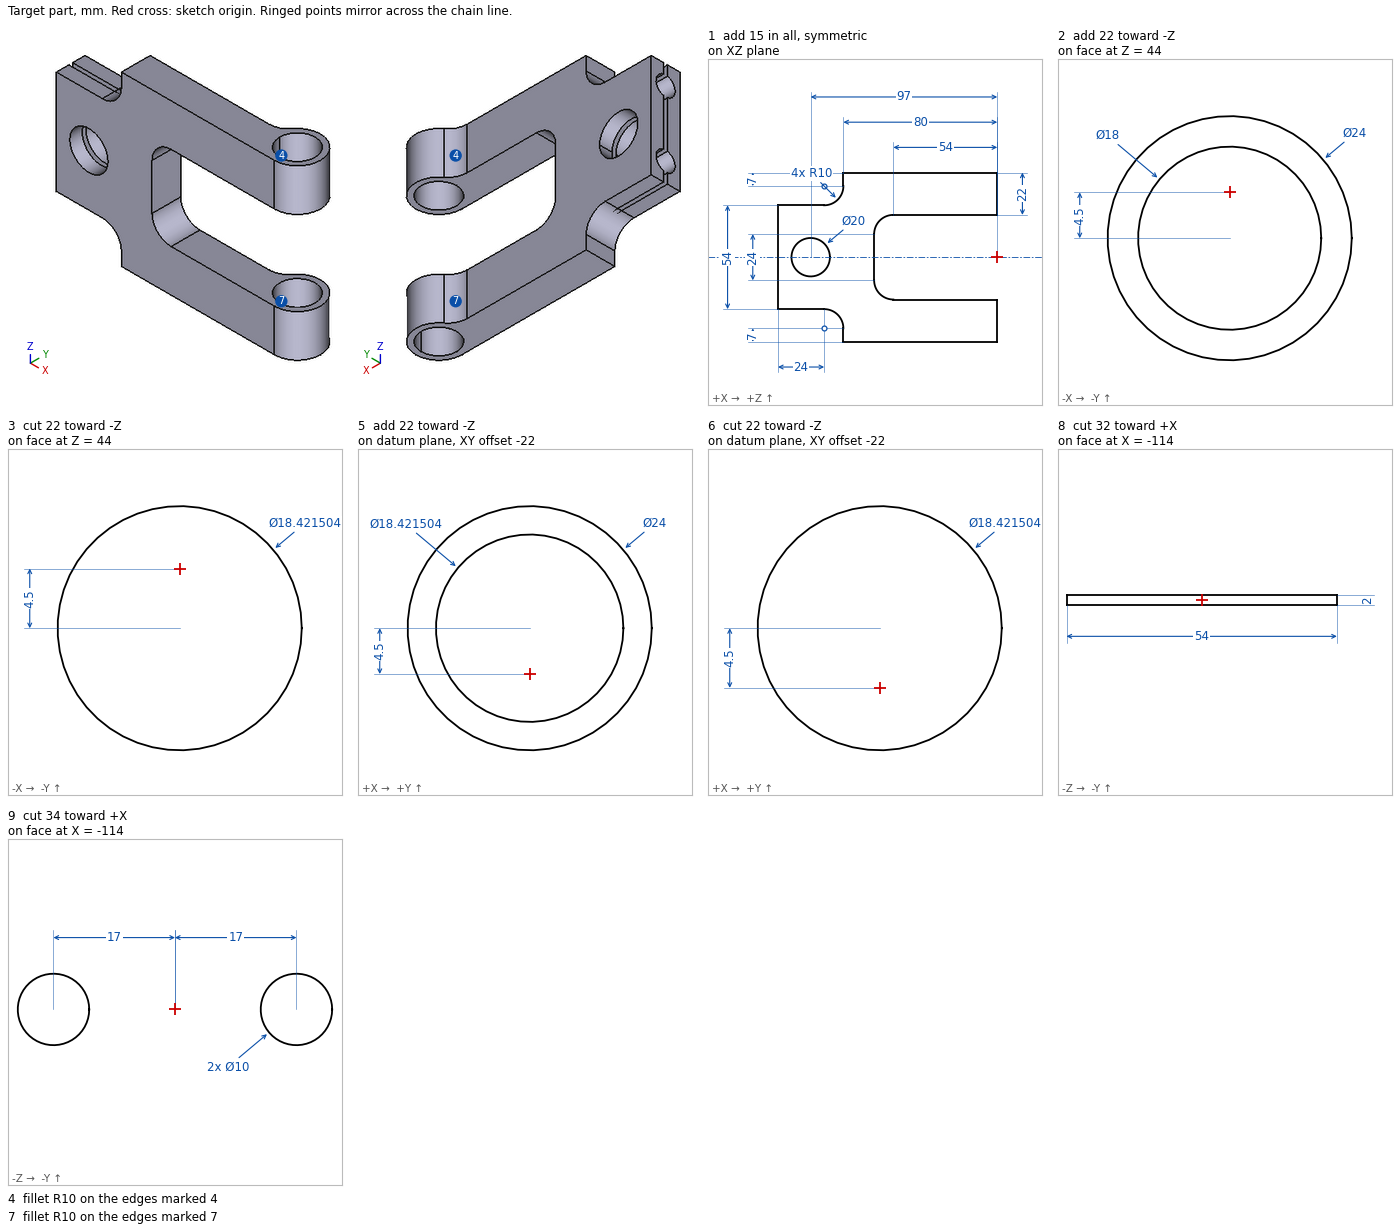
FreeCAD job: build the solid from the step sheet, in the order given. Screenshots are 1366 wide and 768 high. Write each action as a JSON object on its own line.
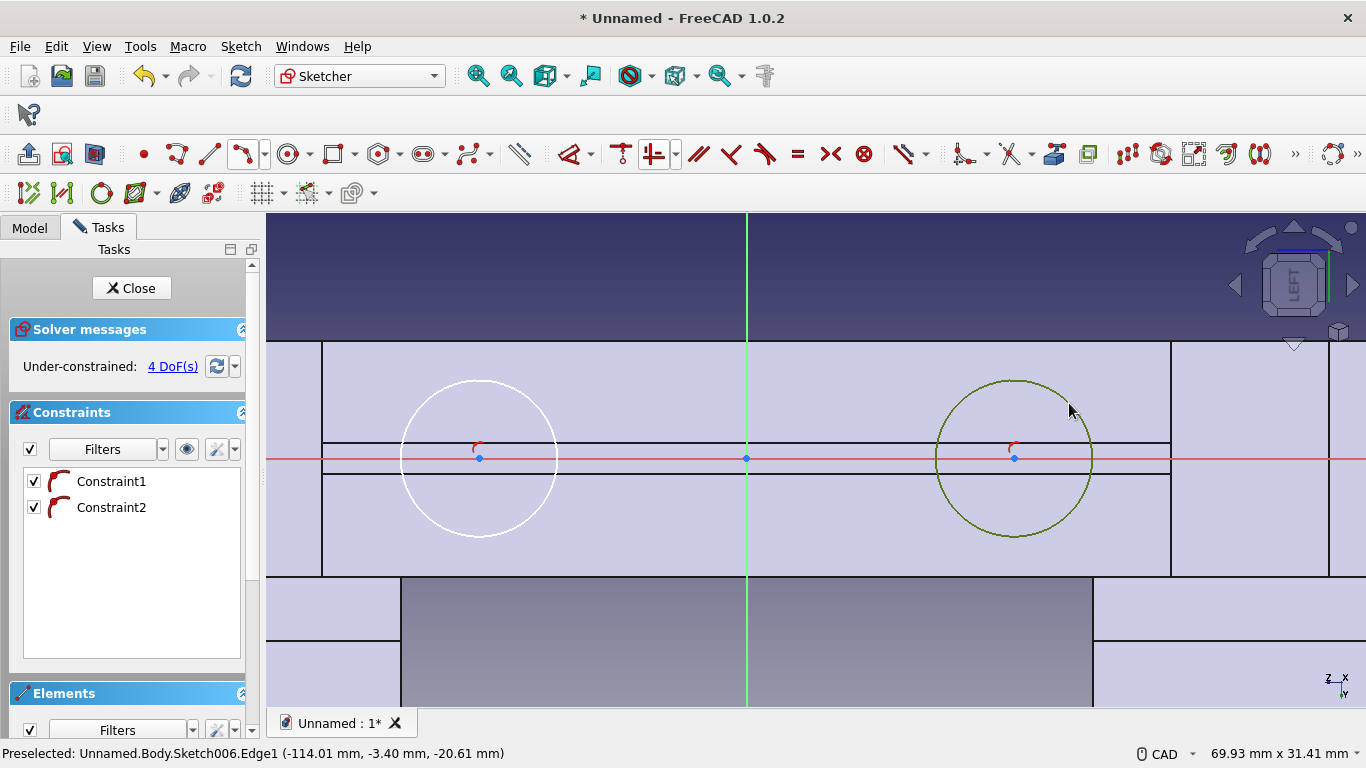
{"action": "left_click", "coordinate": [534, 403]}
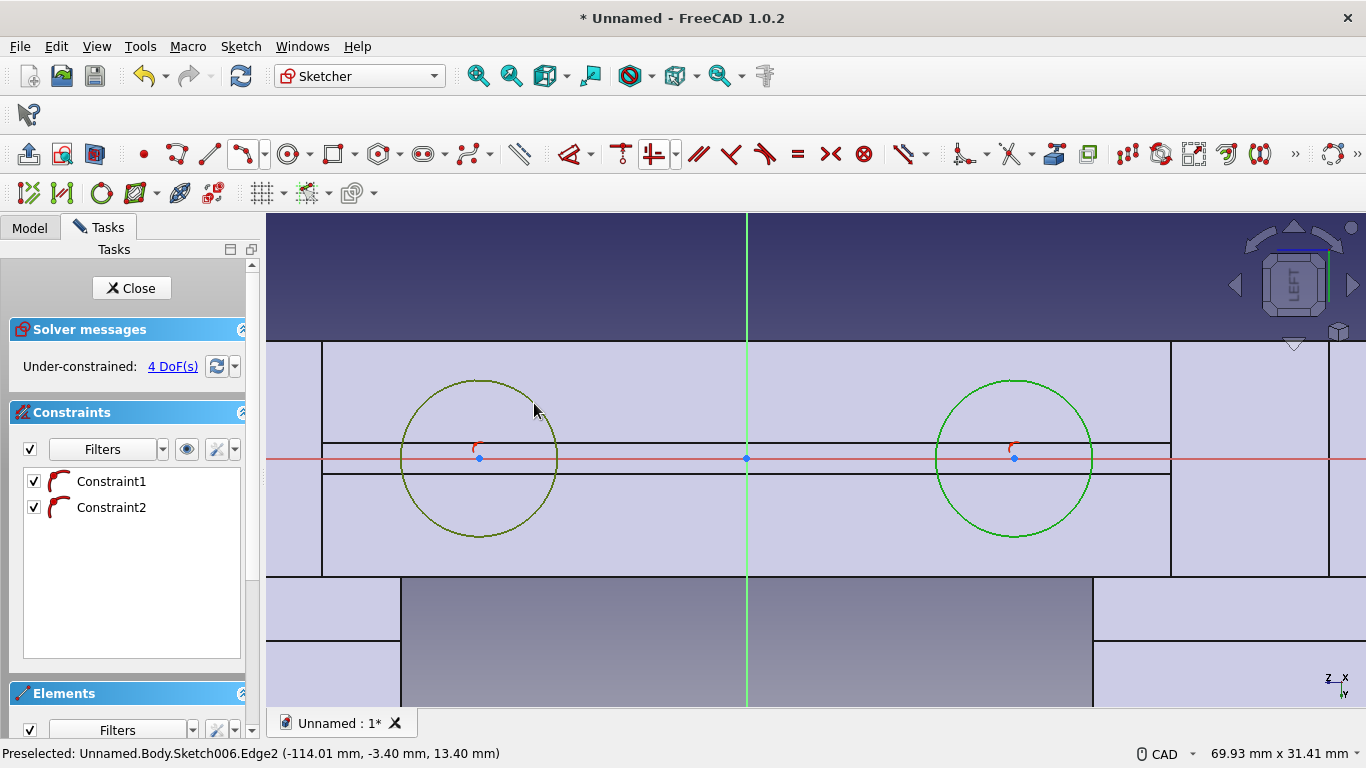
{"action": "left_click", "coordinate": [798, 154]}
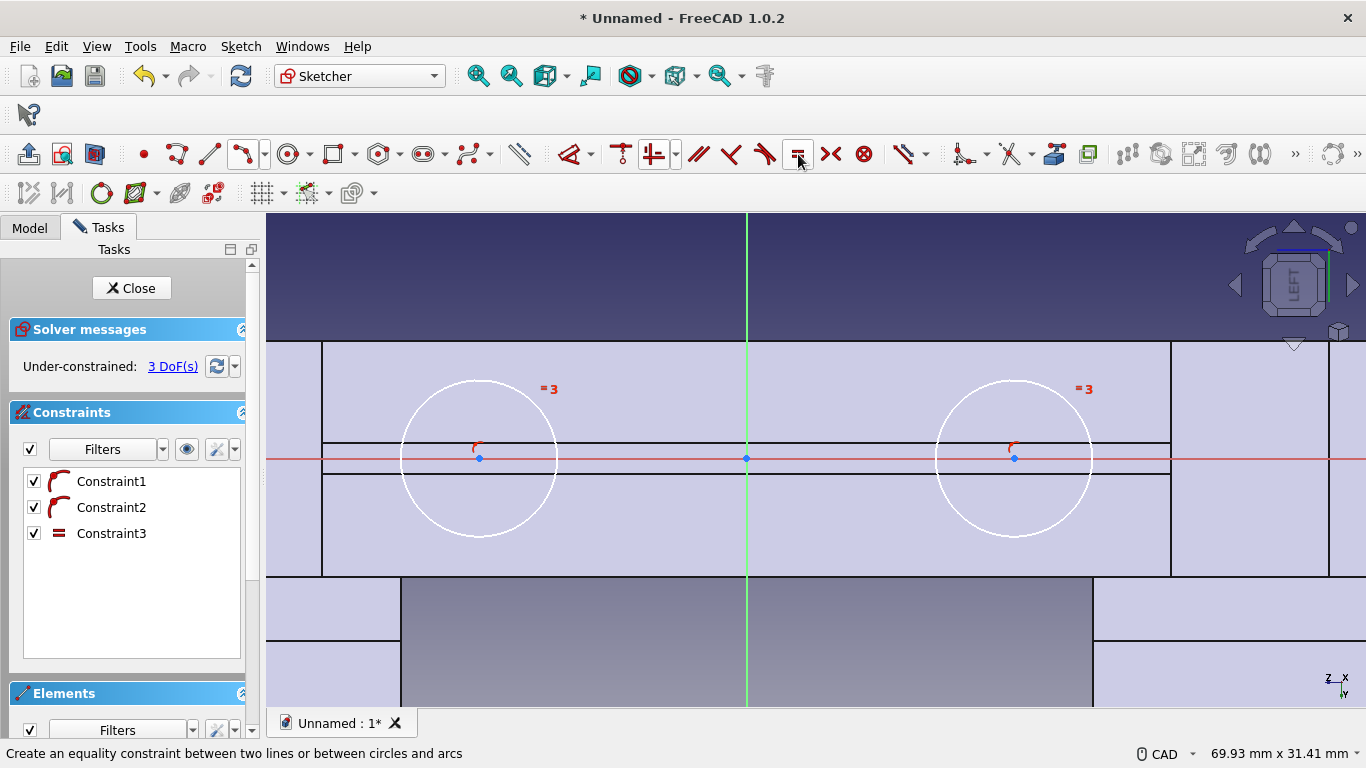
{"action": "left_click", "coordinate": [568, 154]}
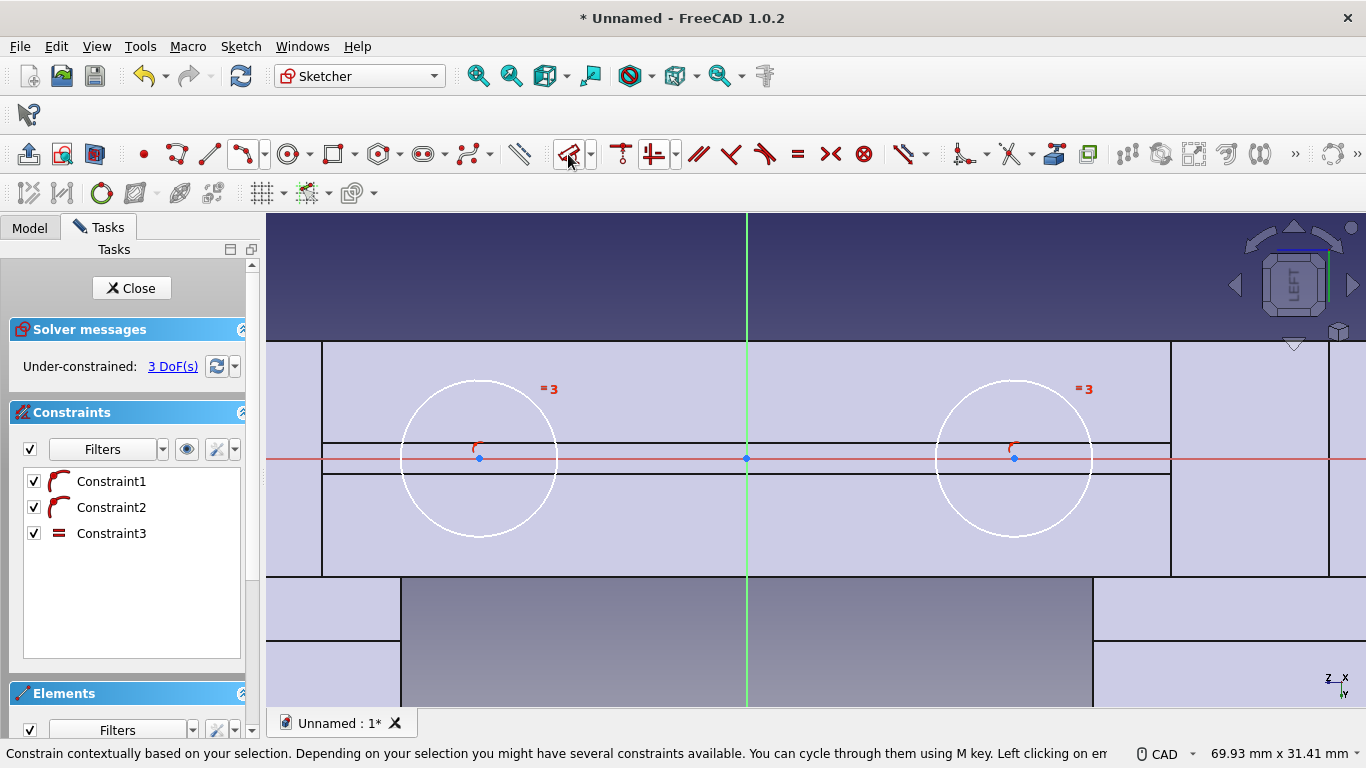
{"action": "left_click", "coordinate": [1069, 403]}
{"action": "left_click", "coordinate": [1092, 380]}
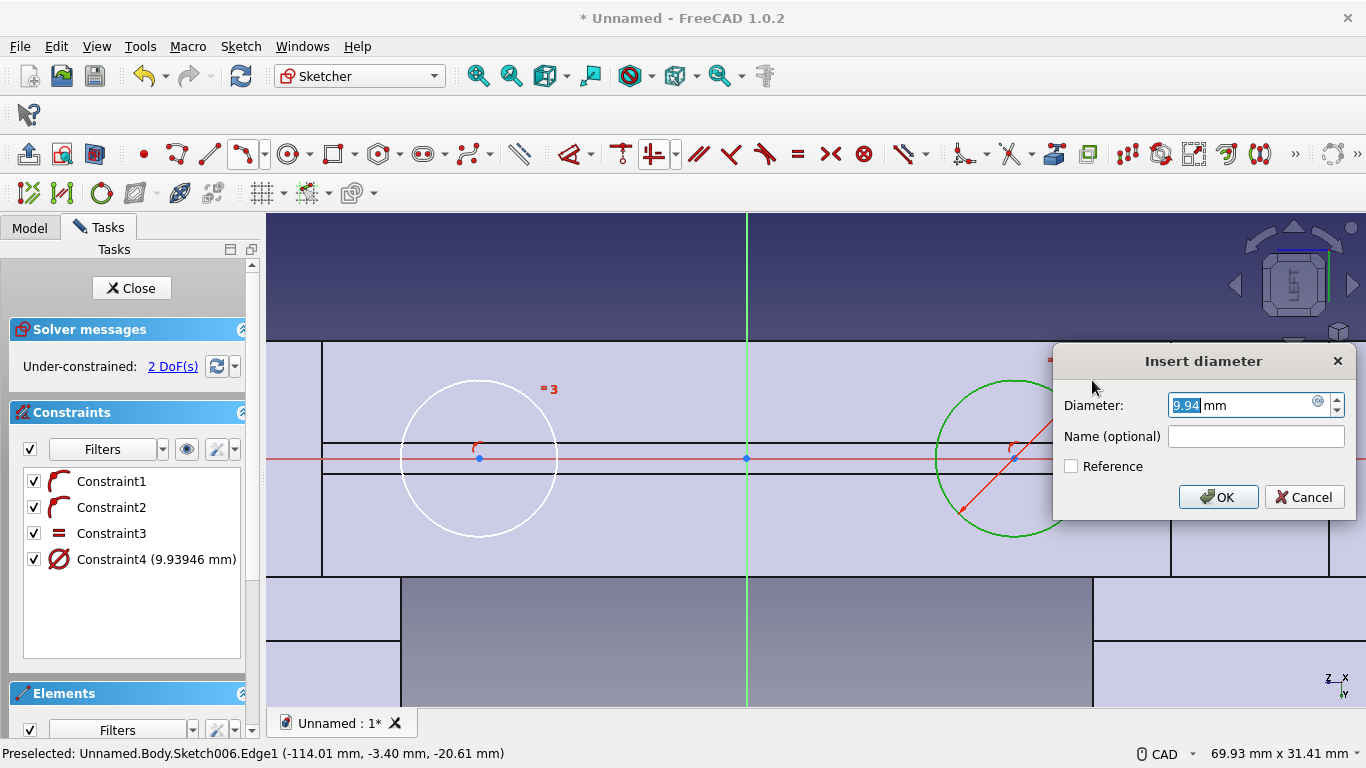
{"action": "type", "text": "10"}
{"action": "key", "text": "Return"}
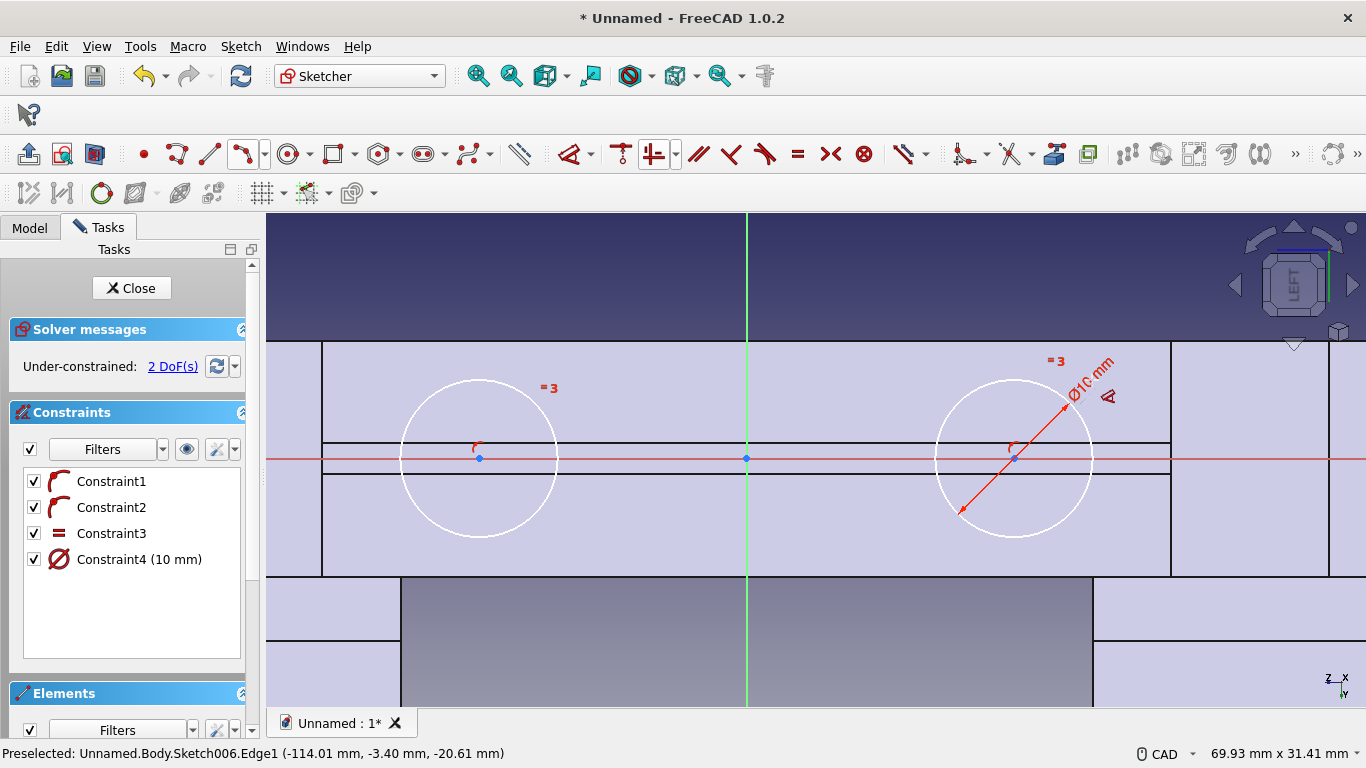
{"action": "left_click", "coordinate": [1014, 459]}
{"action": "left_click", "coordinate": [880, 493]}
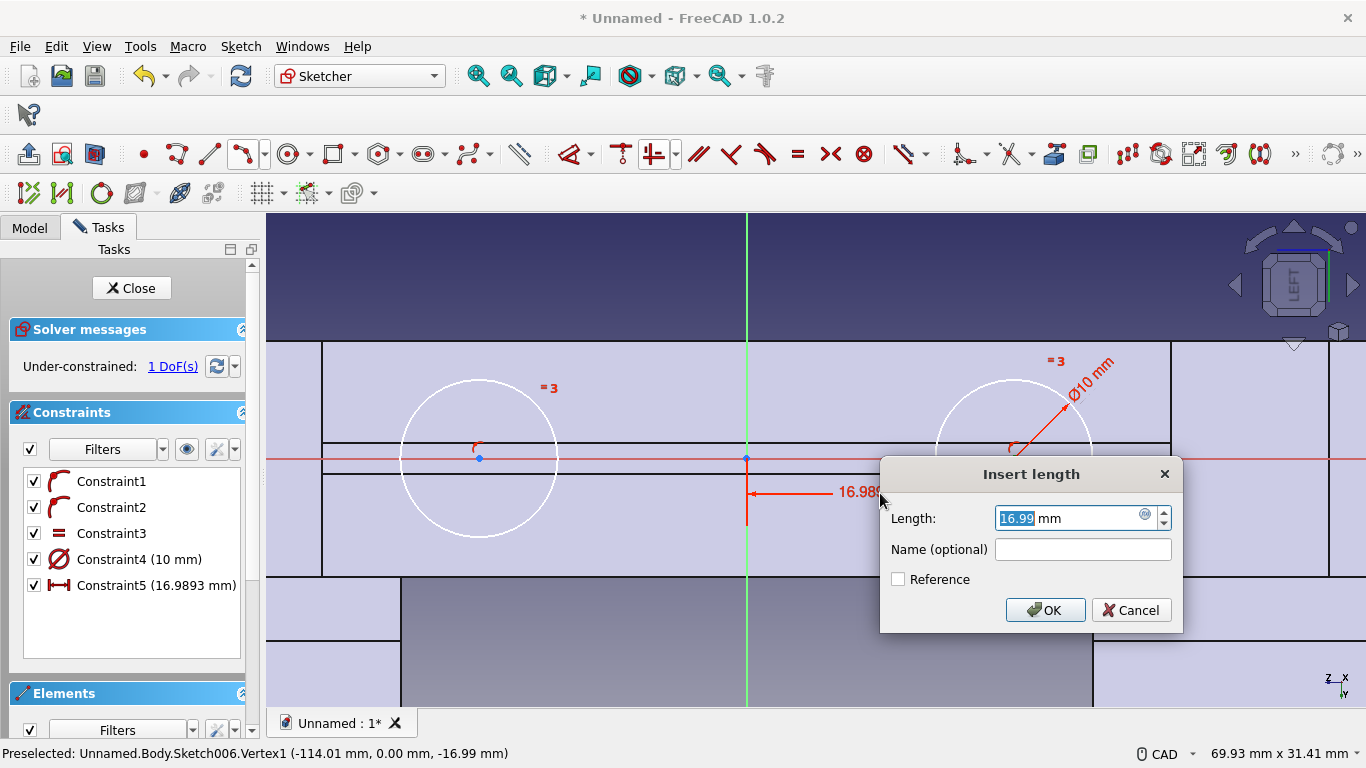
{"action": "type", "text": "17"}
{"action": "key", "text": "Return"}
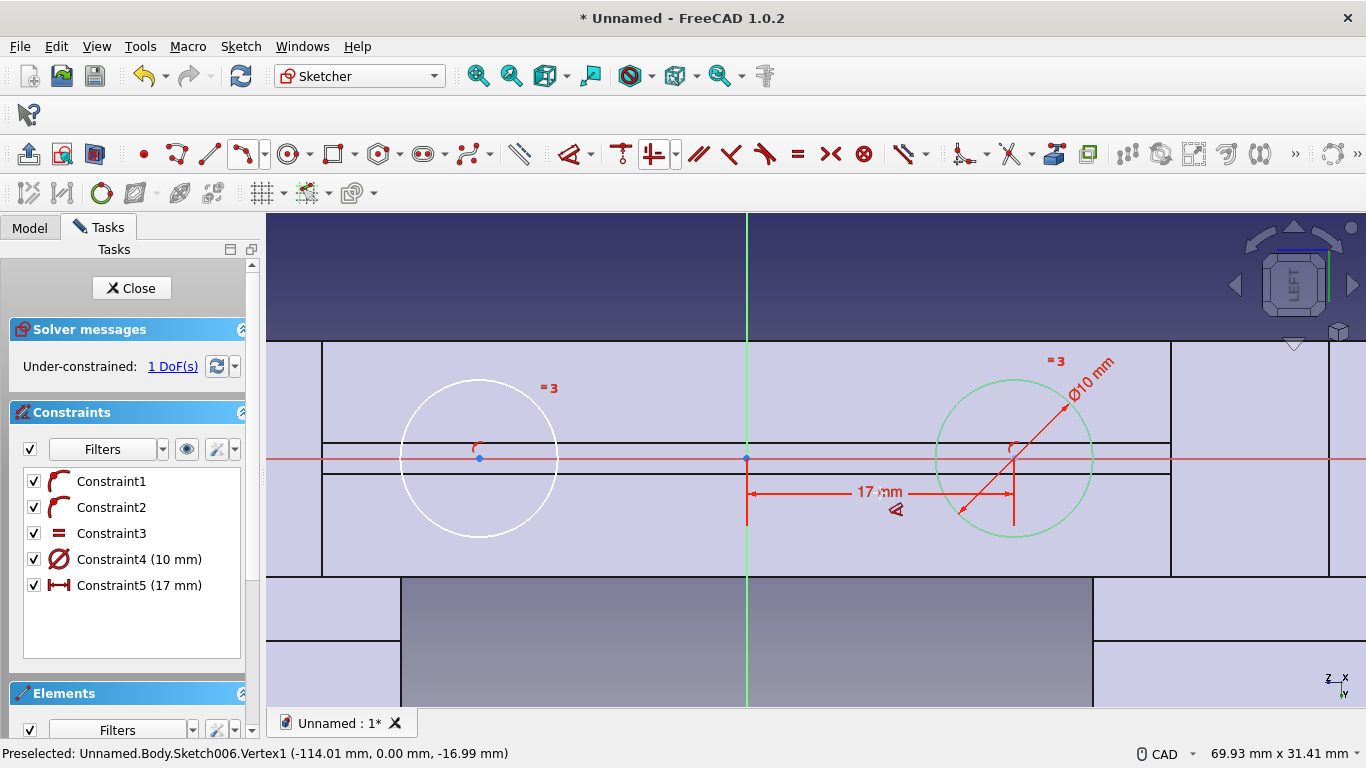
{"action": "left_click", "coordinate": [479, 459]}
{"action": "left_click", "coordinate": [613, 493]}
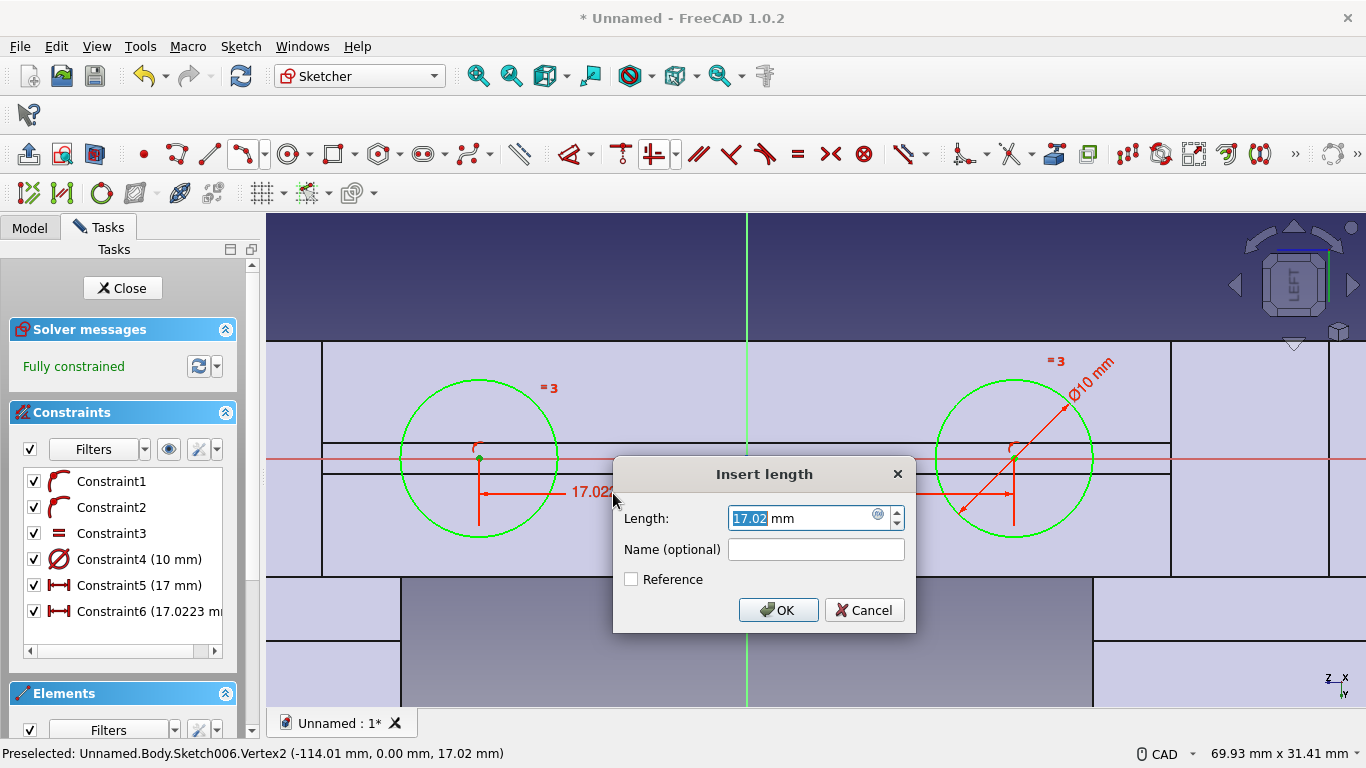
{"action": "type", "text": "17"}
{"action": "key", "text": "Return"}
{"action": "key", "text": "Escape"}